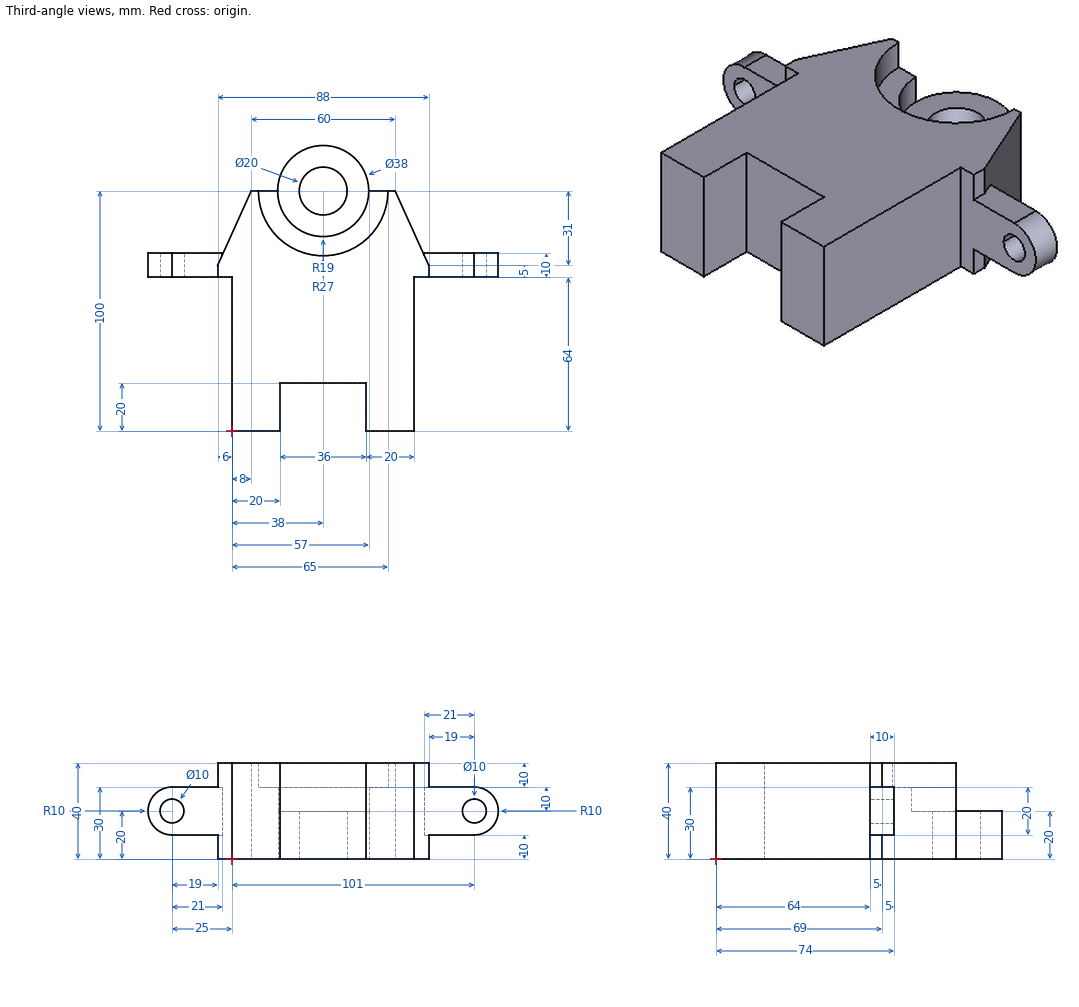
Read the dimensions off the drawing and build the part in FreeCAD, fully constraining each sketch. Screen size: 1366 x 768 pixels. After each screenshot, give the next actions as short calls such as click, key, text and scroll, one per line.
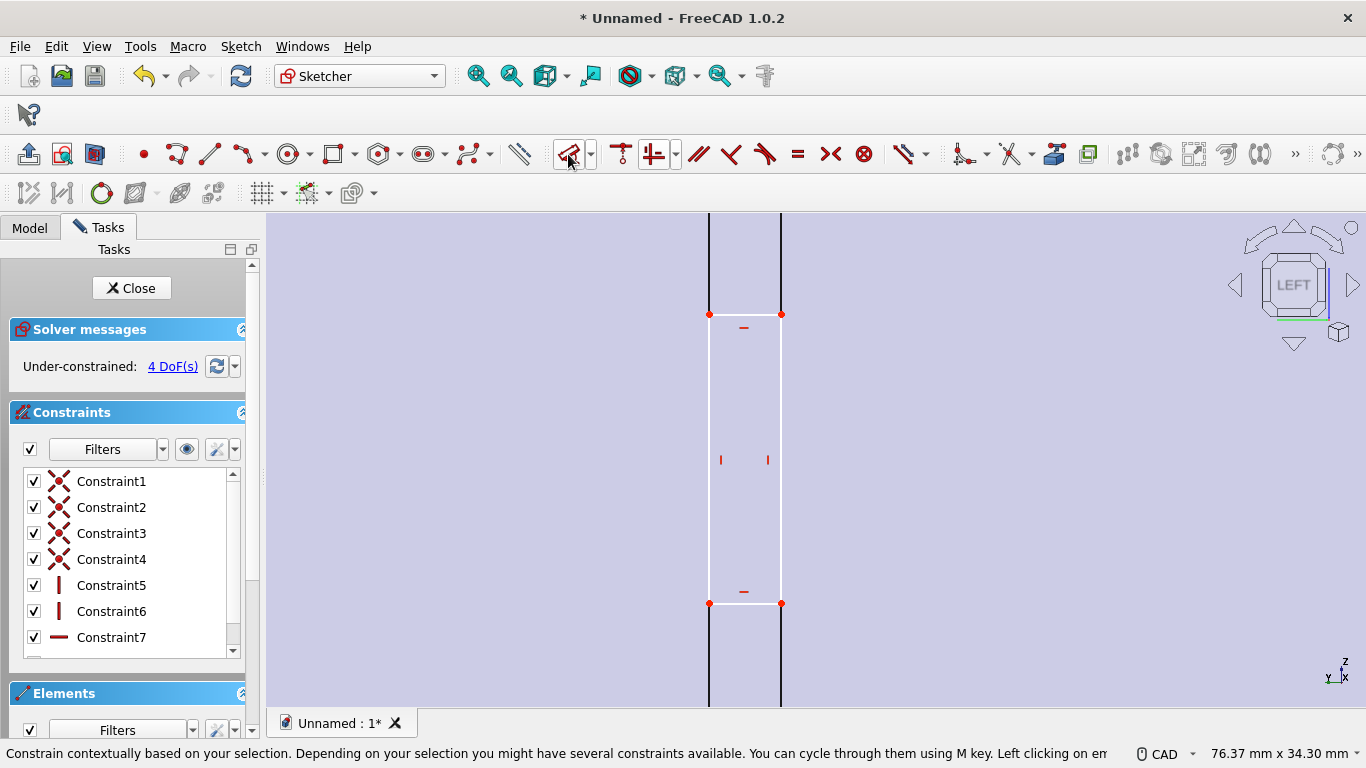
click(731, 604)
click(745, 638)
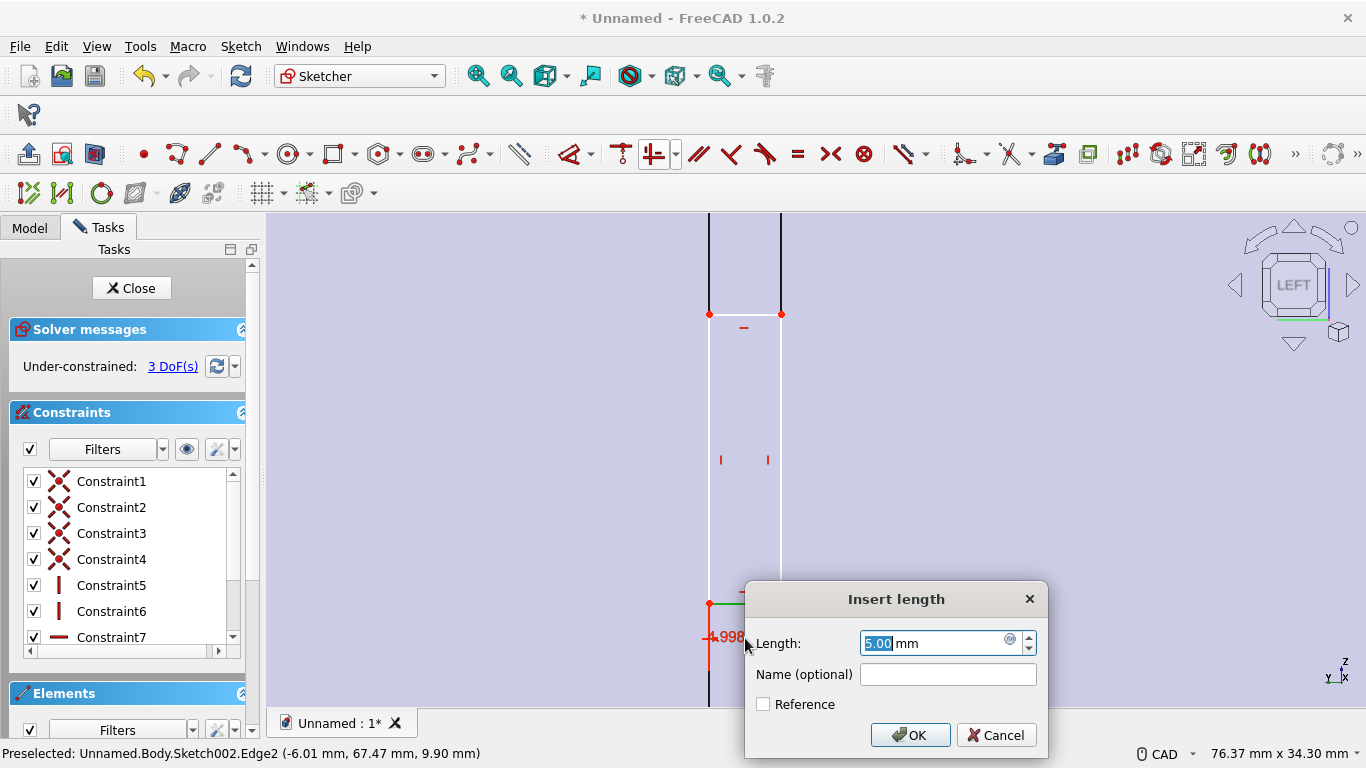
text(5)
key(Return)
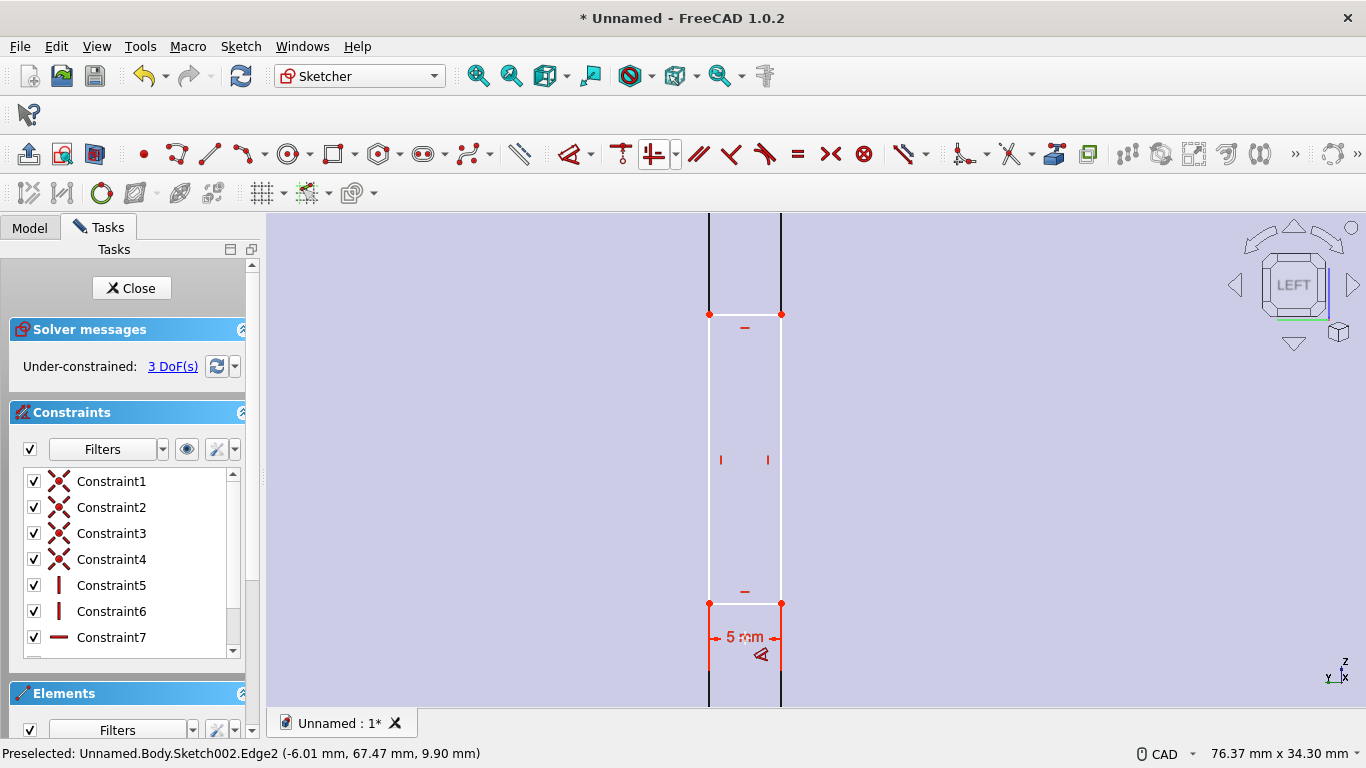
click(709, 402)
click(675, 460)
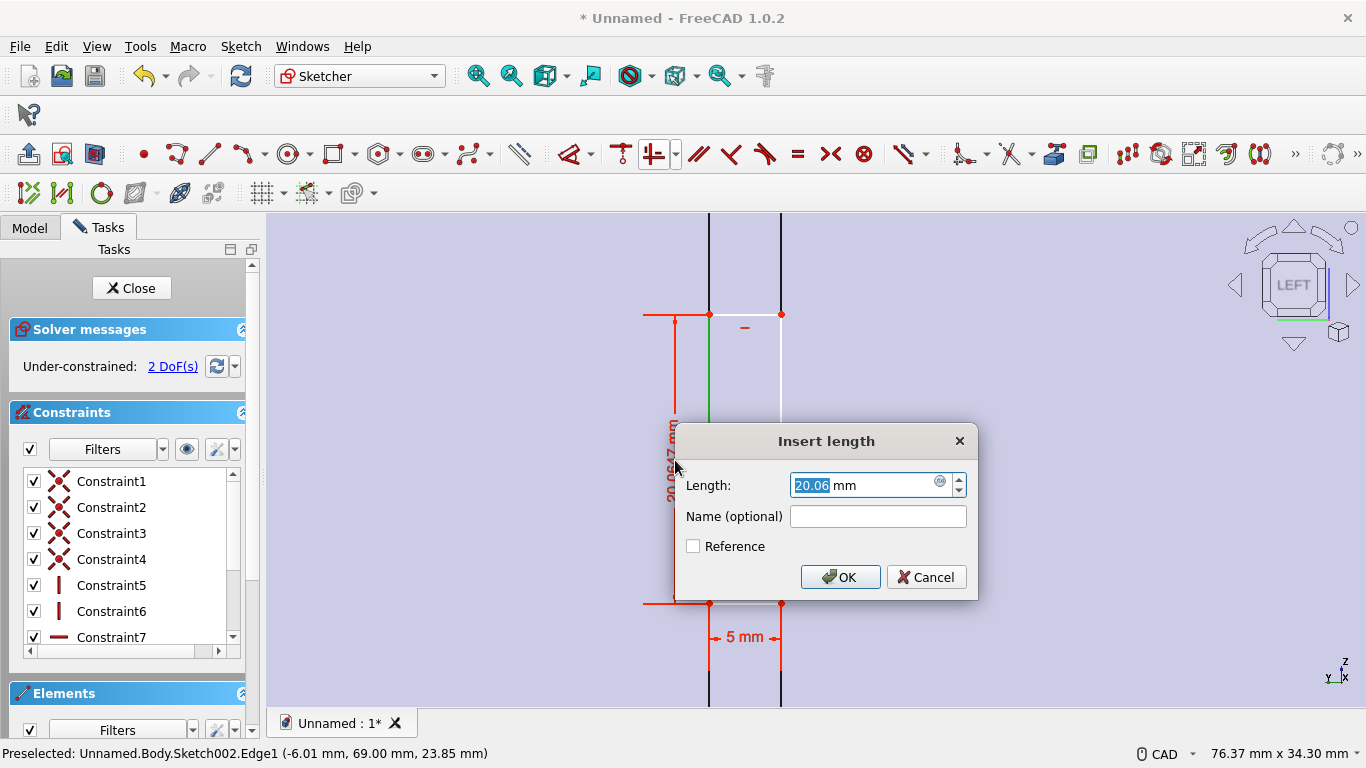
text(20)
key(Return)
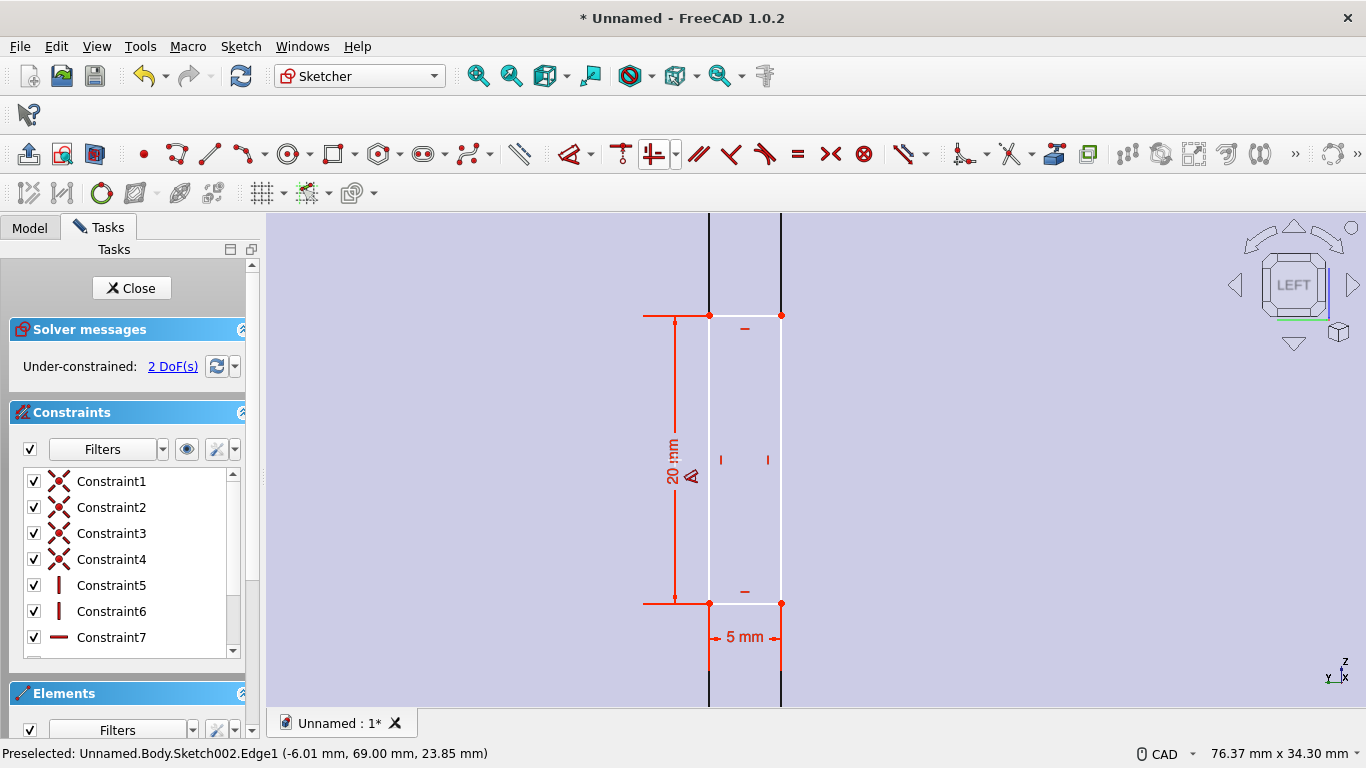
click(709, 316)
click(955, 282)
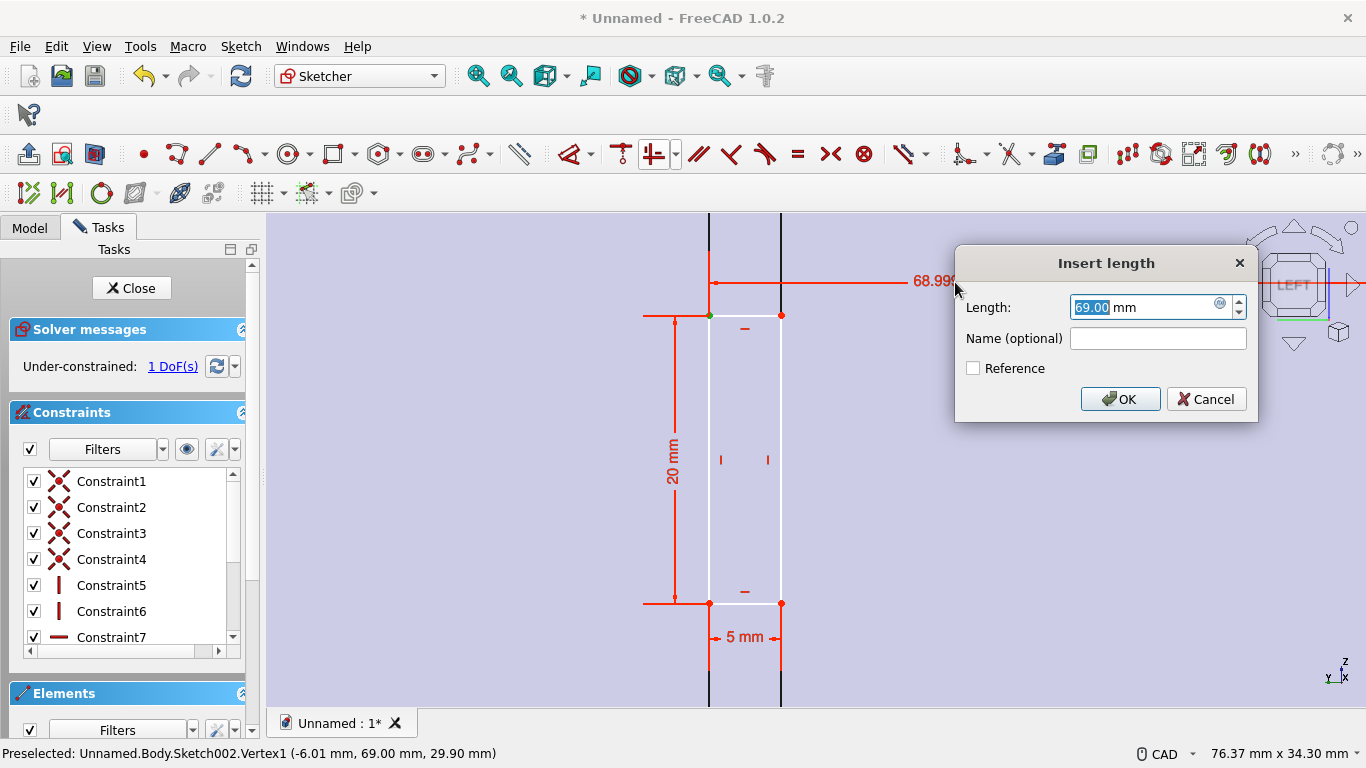
text(69)
key(Return)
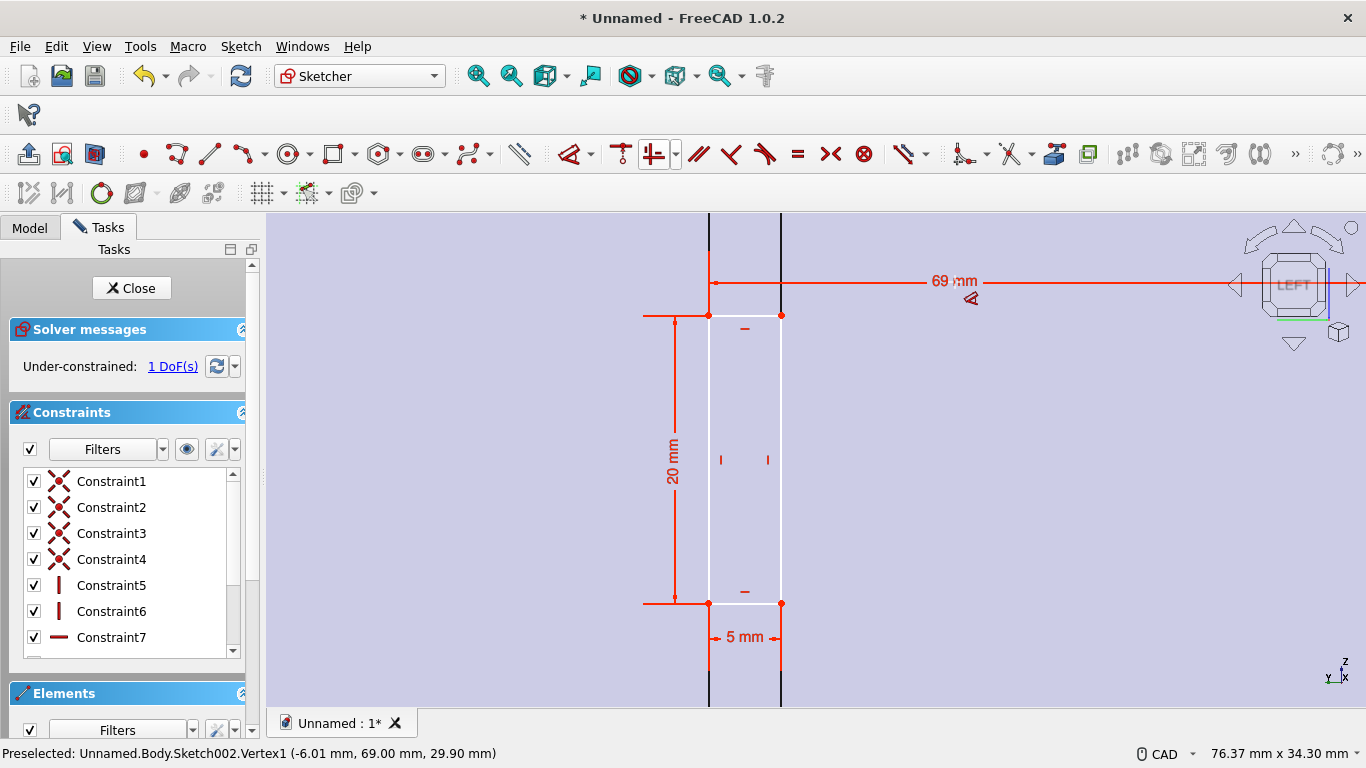
click(709, 316)
click(675, 497)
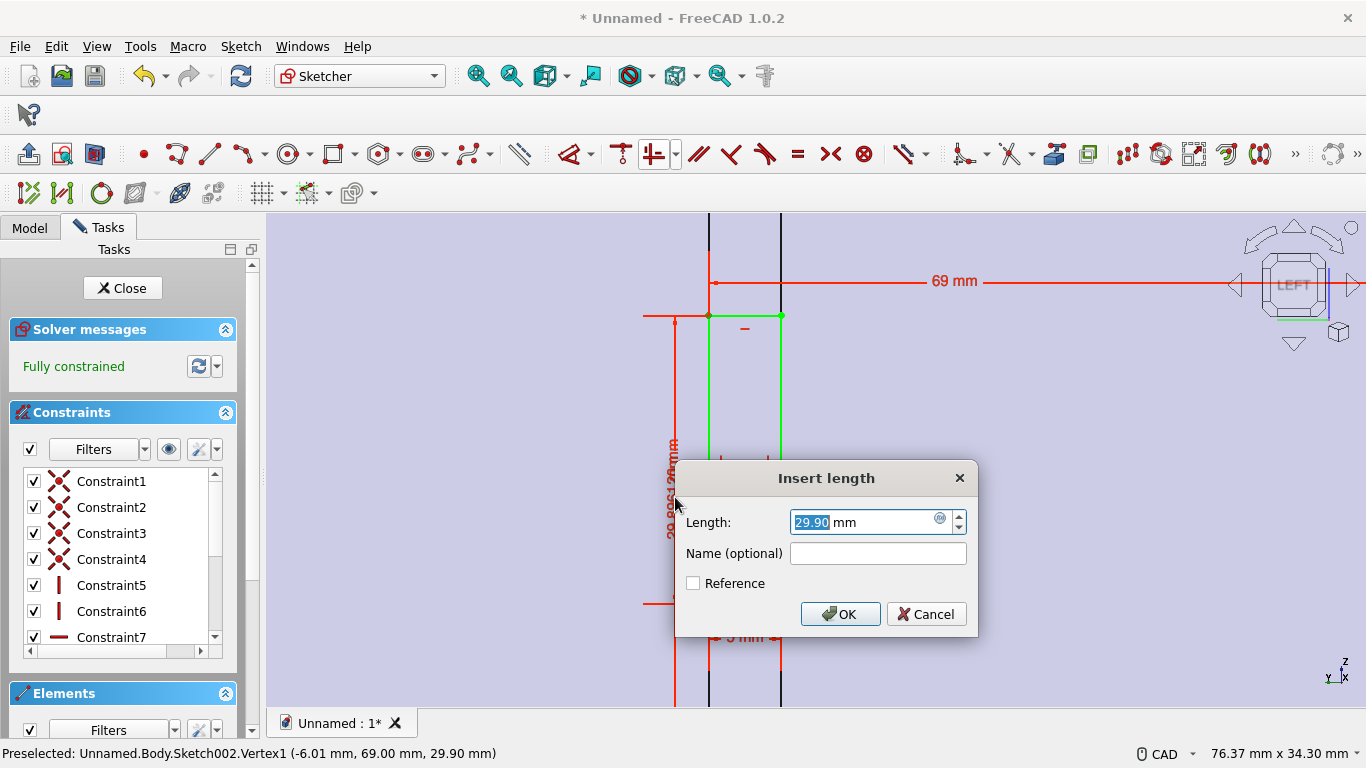
text(30)
key(Return)
key(Escape)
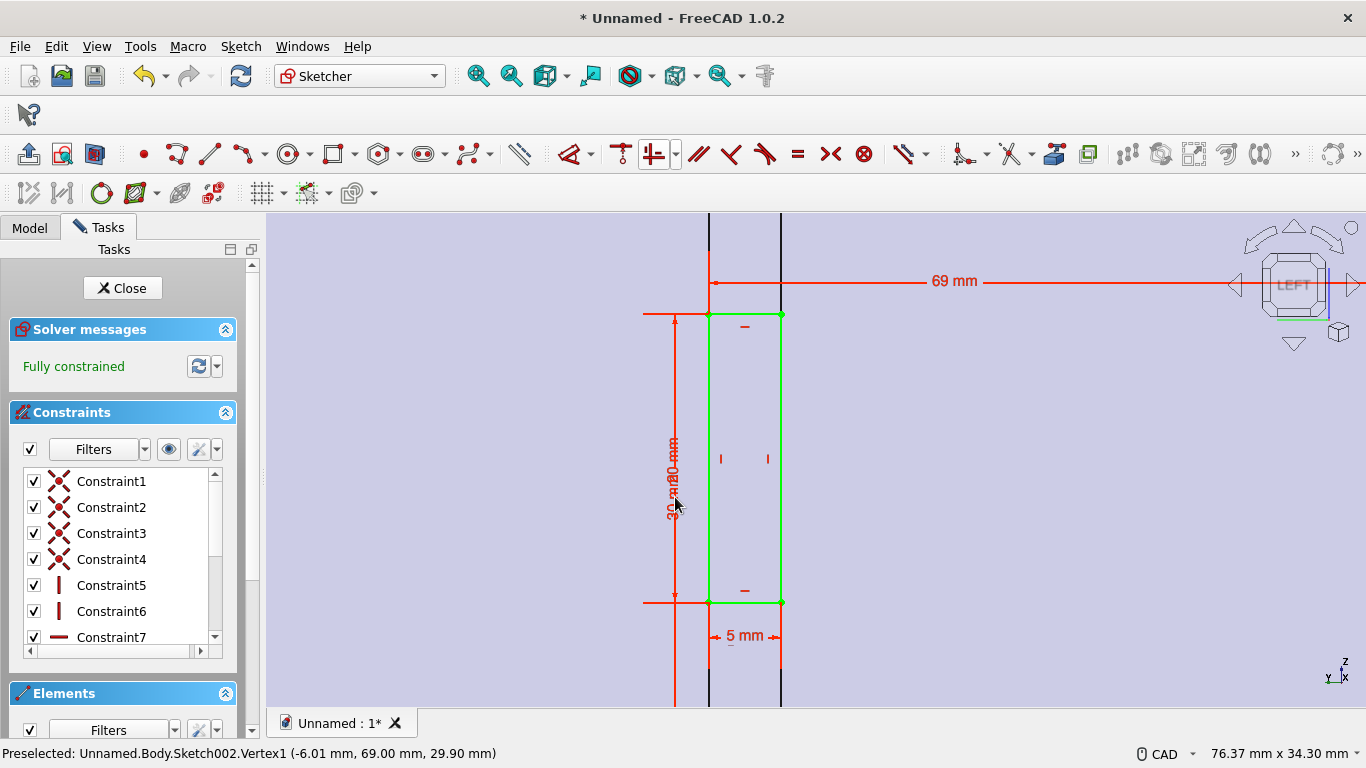
click(123, 288)